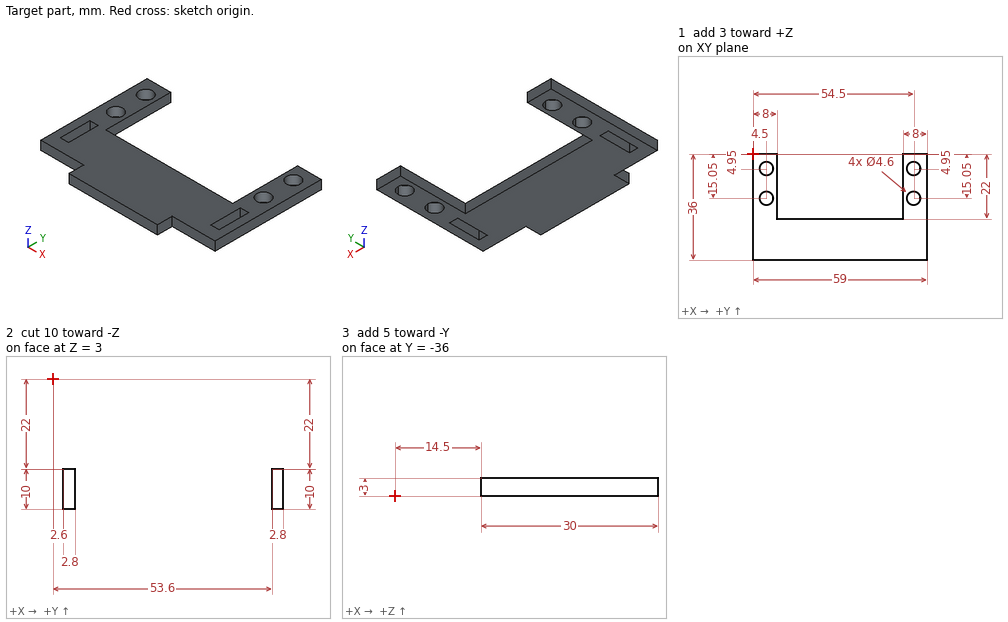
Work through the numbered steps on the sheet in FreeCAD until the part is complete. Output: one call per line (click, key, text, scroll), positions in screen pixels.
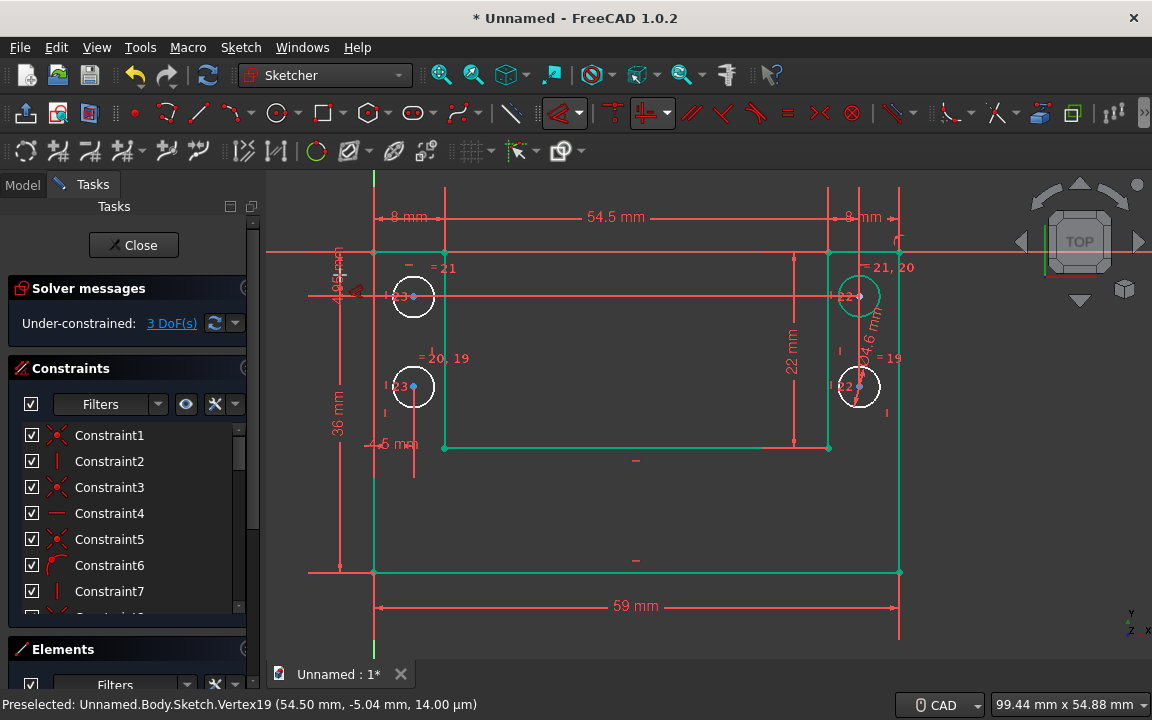
click(414, 297)
click(472, 275)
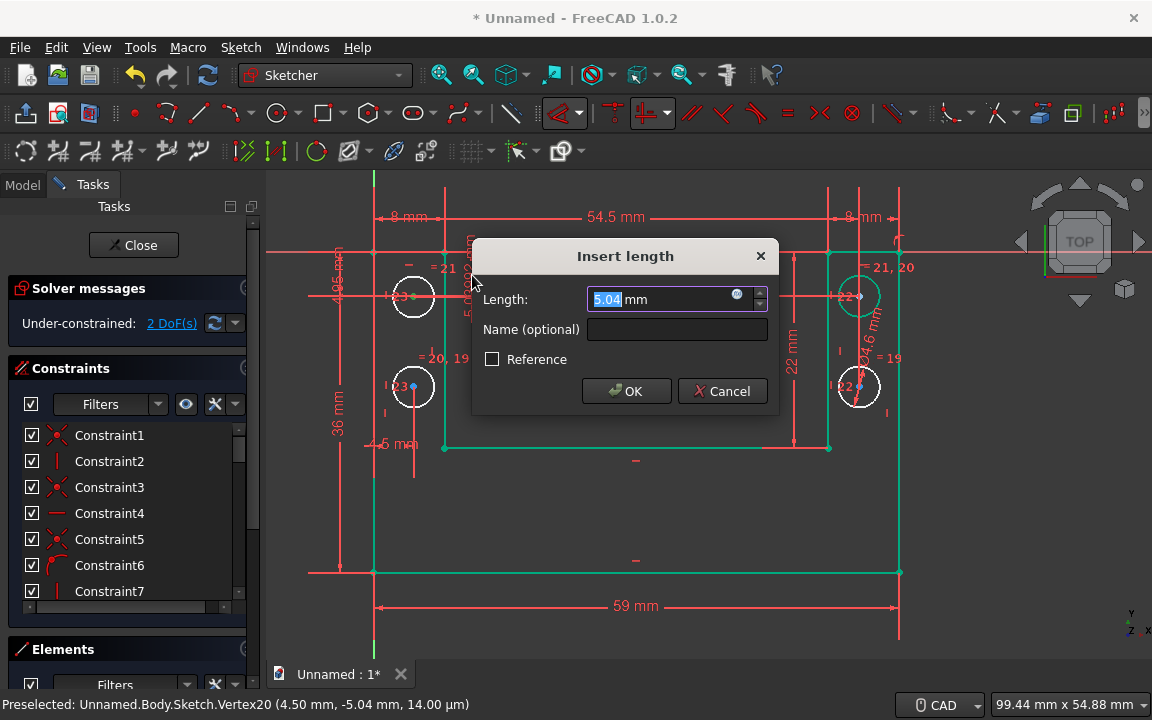
text(4.95)
key(Return)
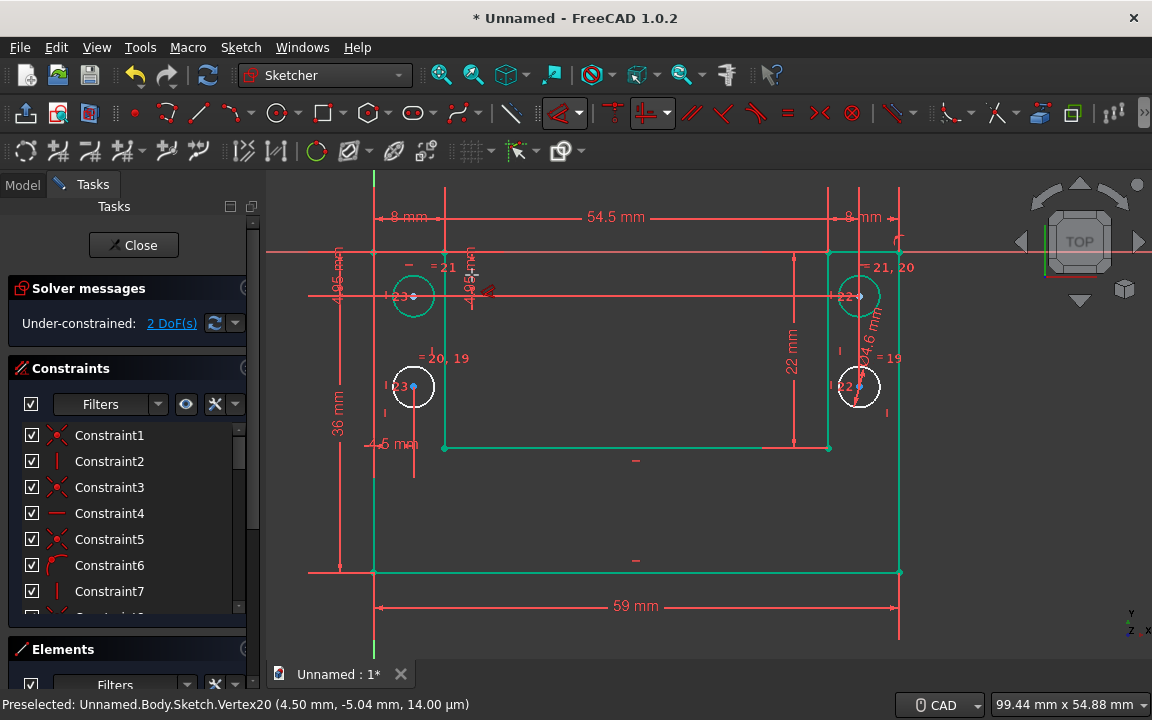
click(859, 387)
click(340, 320)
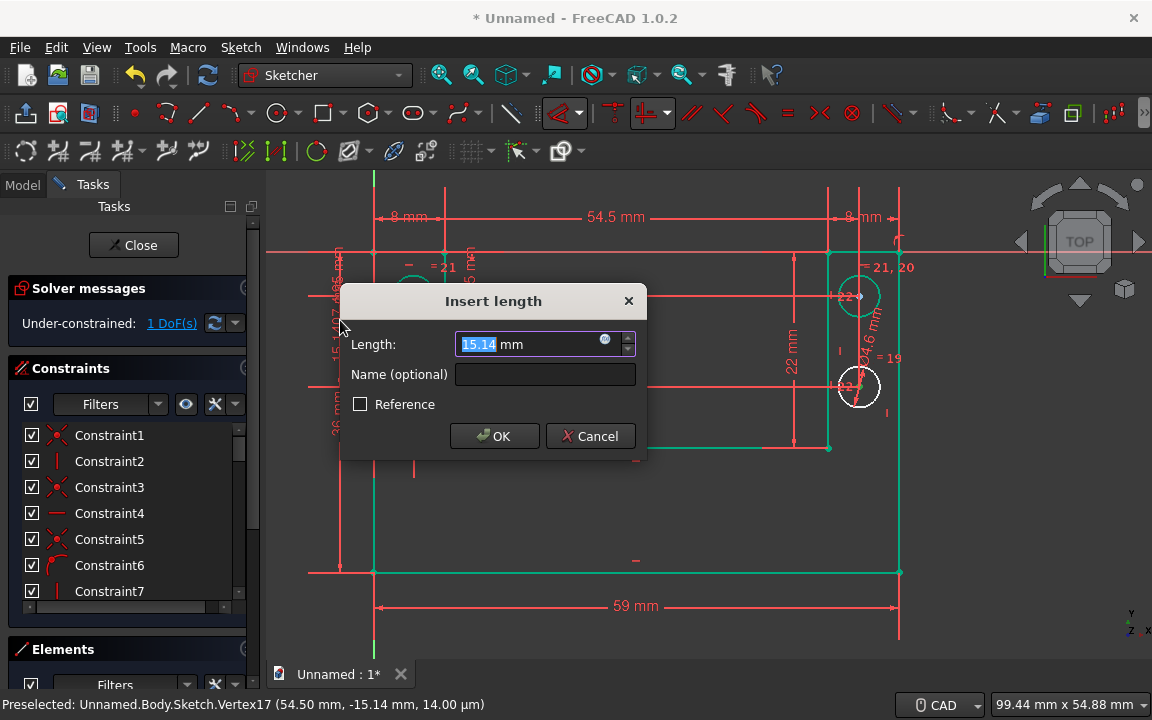
text(15.05)
key(Return)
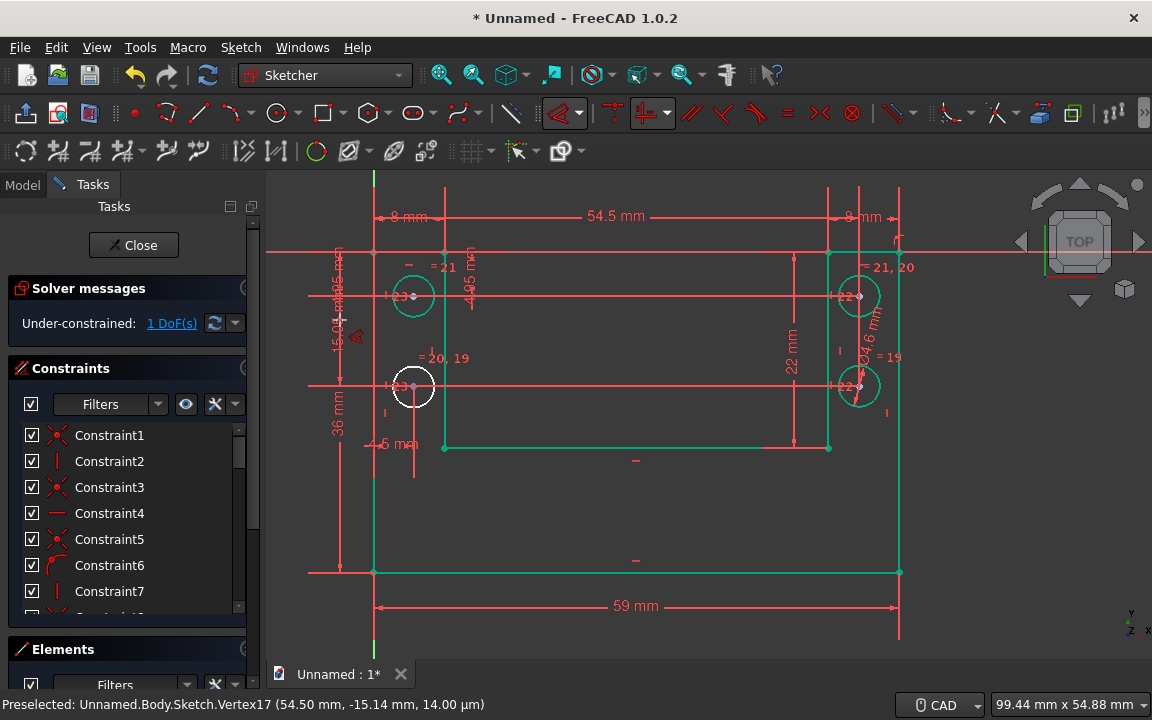
click(414, 387)
click(340, 351)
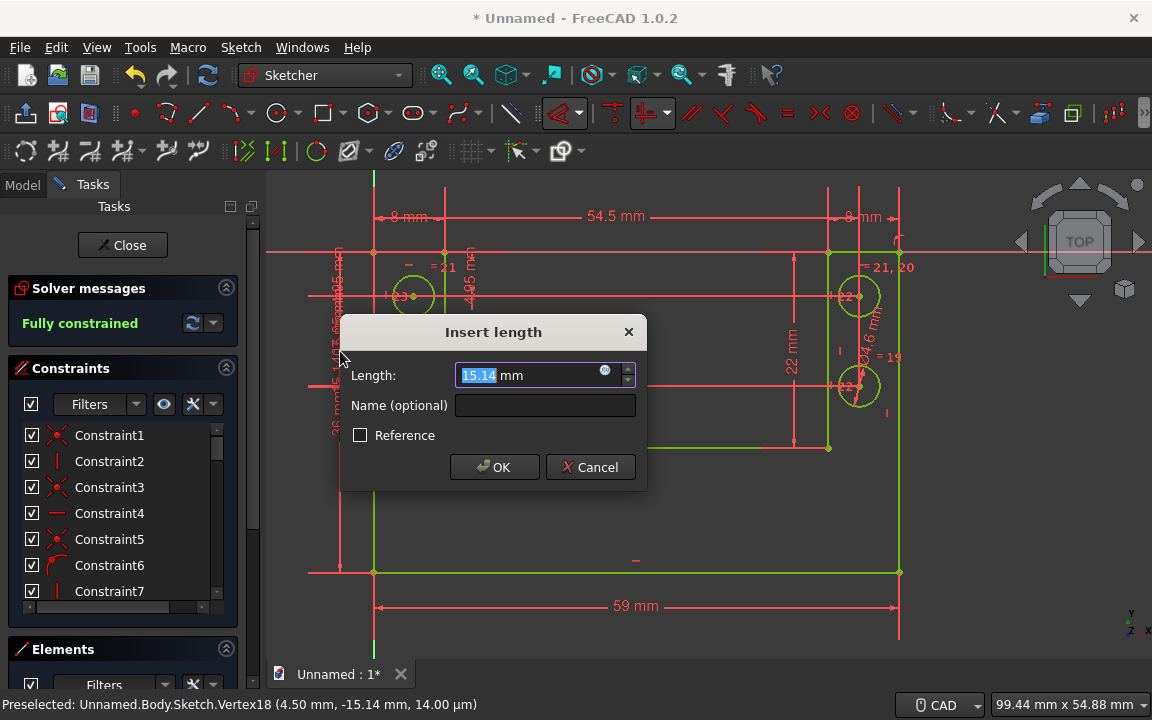
text(15.05)
key(Return)
key(Escape)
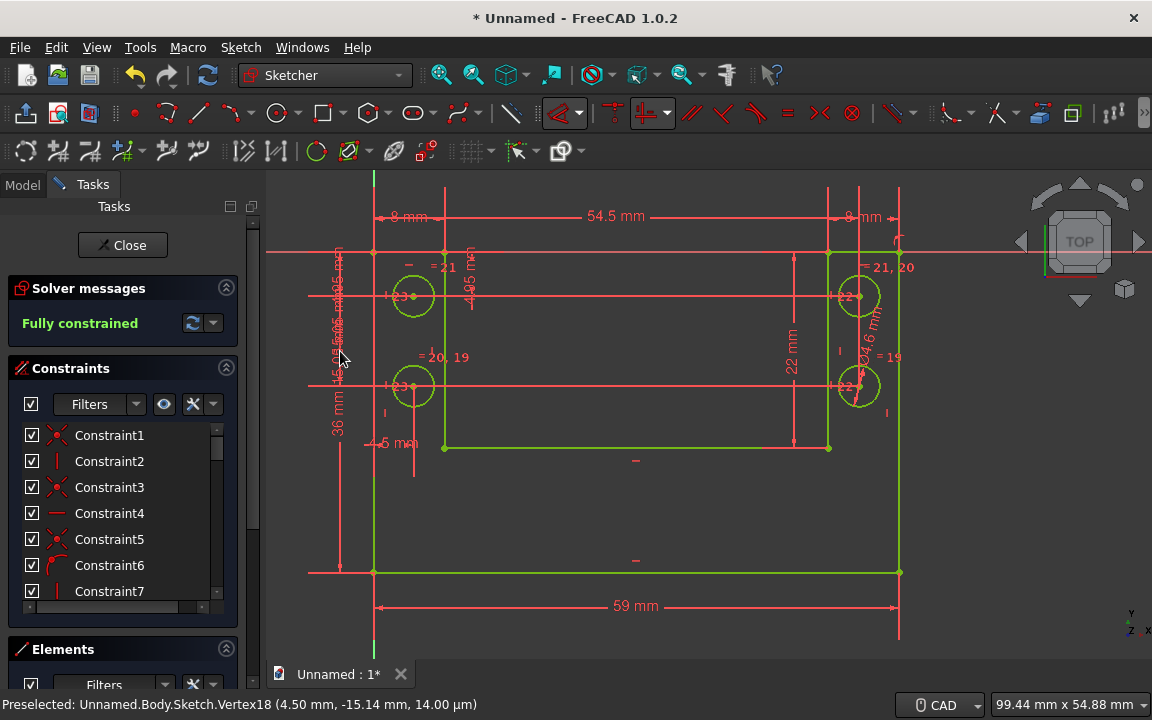
click(123, 245)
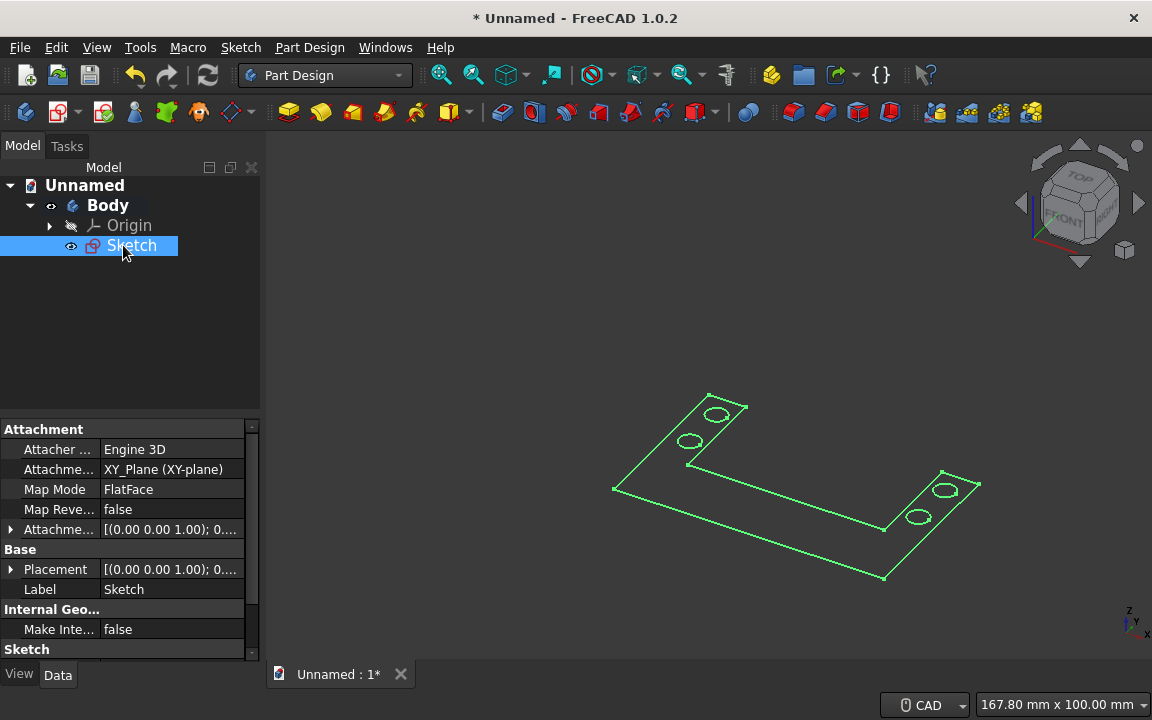
click(290, 112)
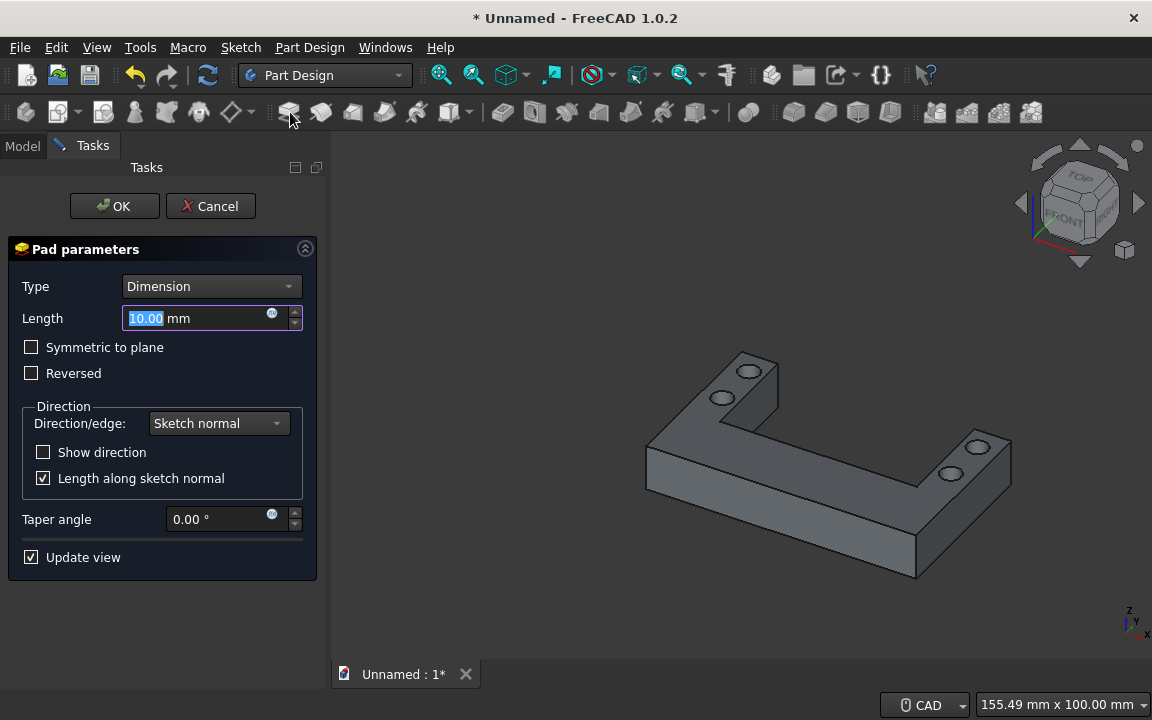
text(3)
key(Tab)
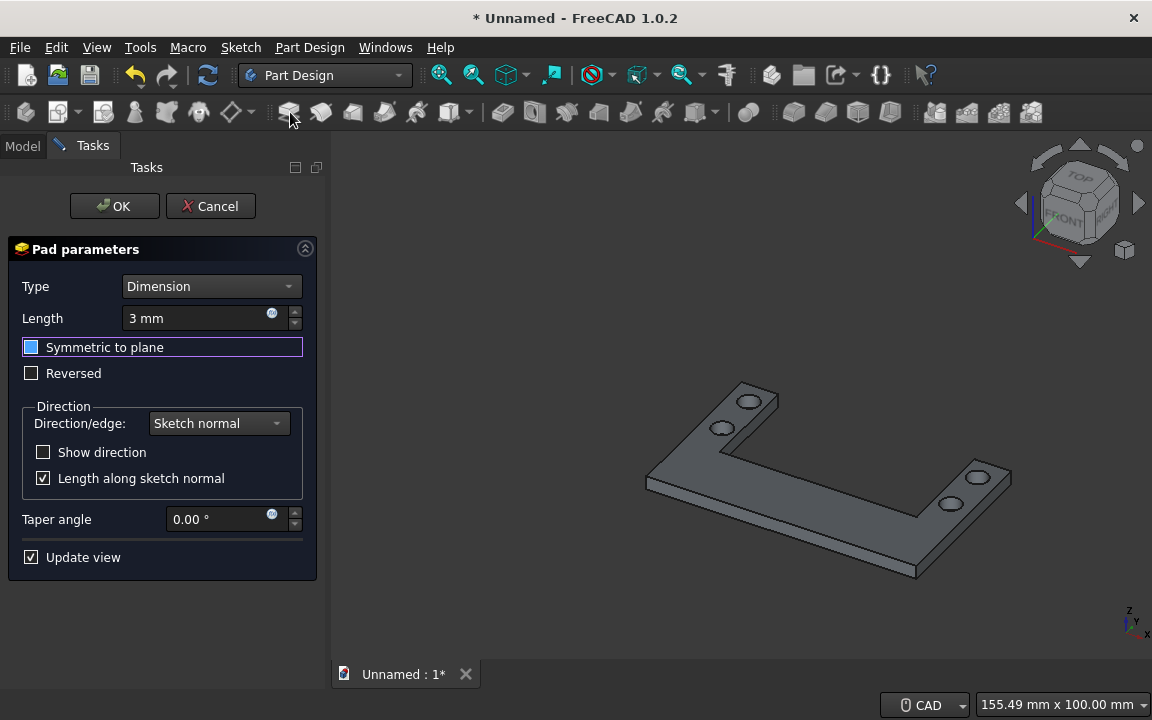
click(115, 206)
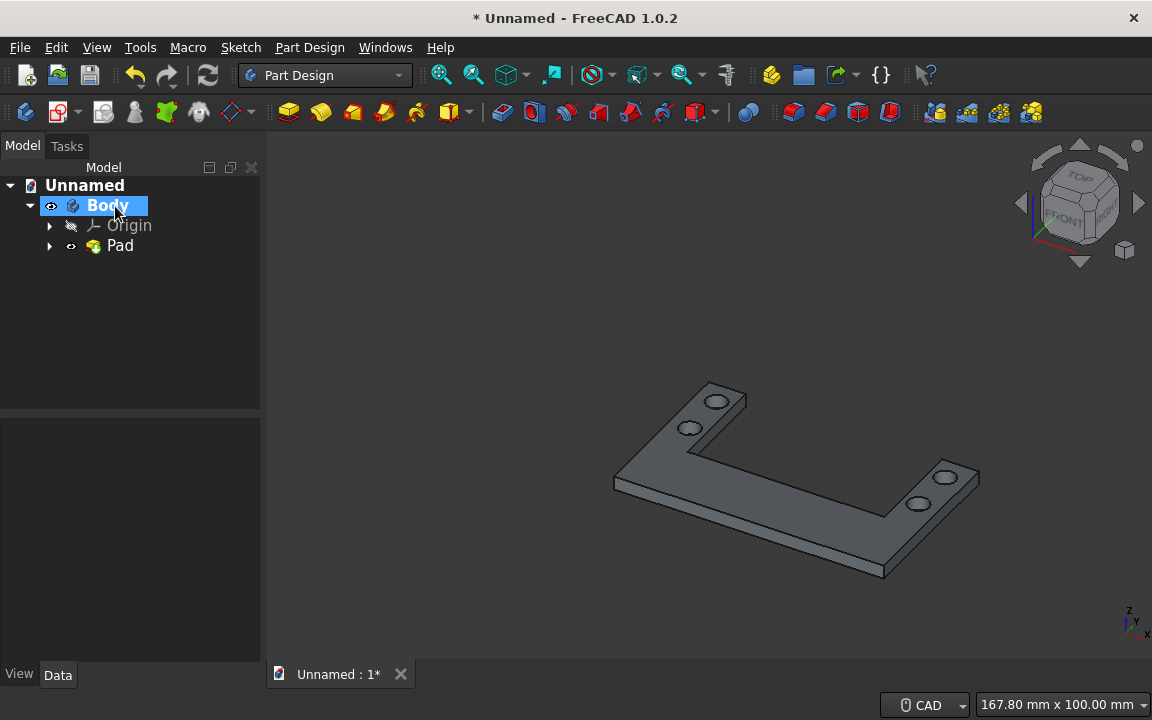
key(v)
key(f)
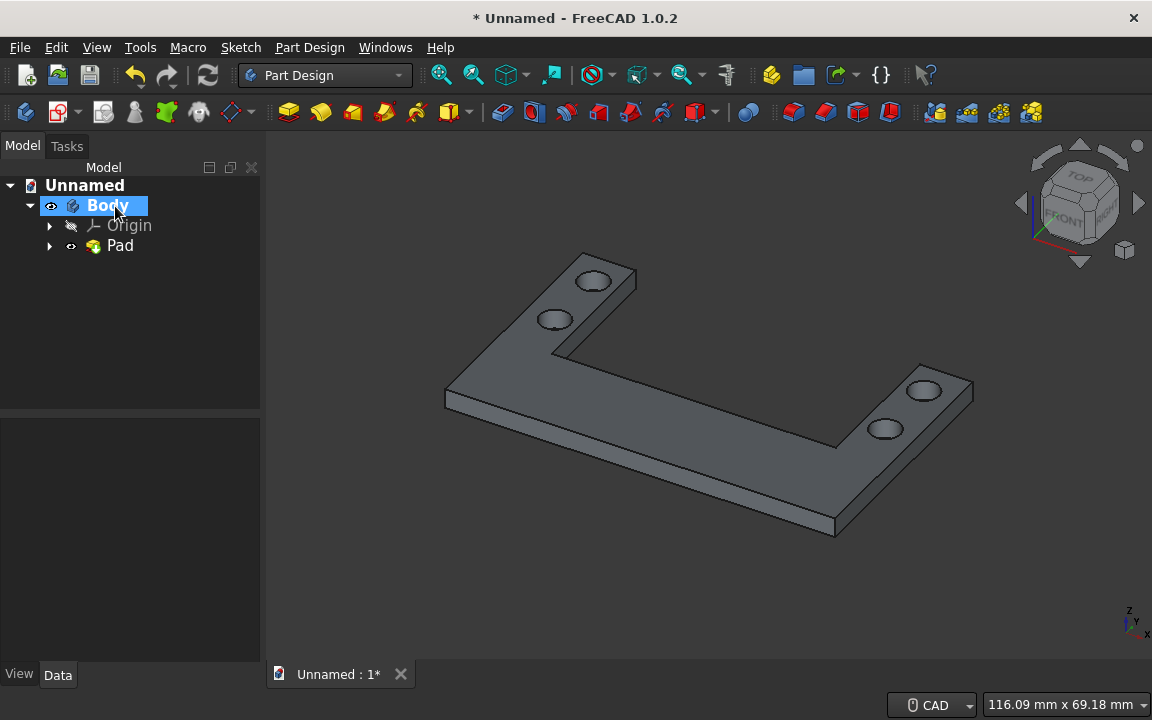
click(781, 461)